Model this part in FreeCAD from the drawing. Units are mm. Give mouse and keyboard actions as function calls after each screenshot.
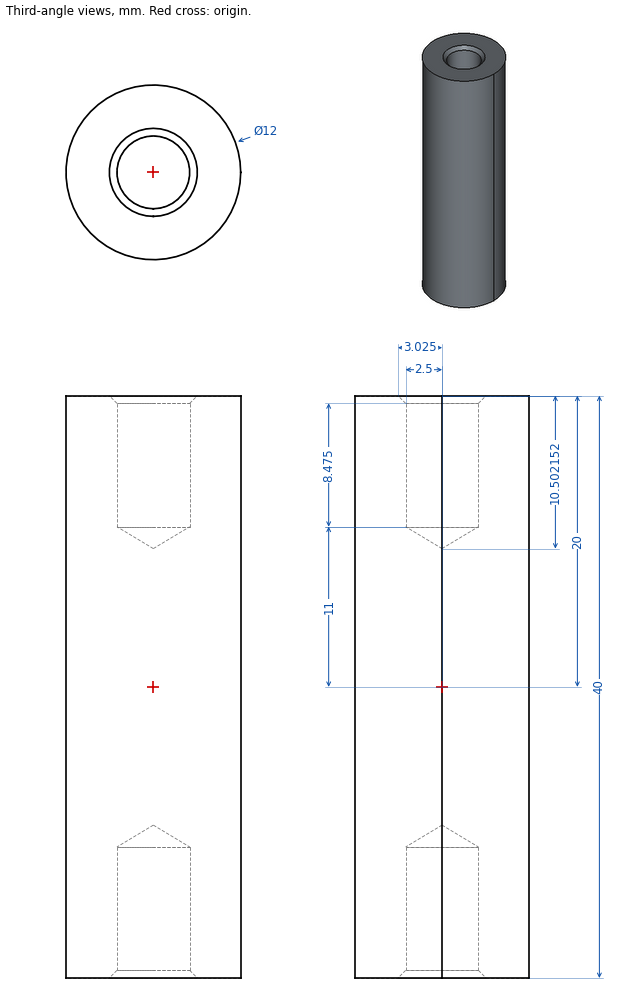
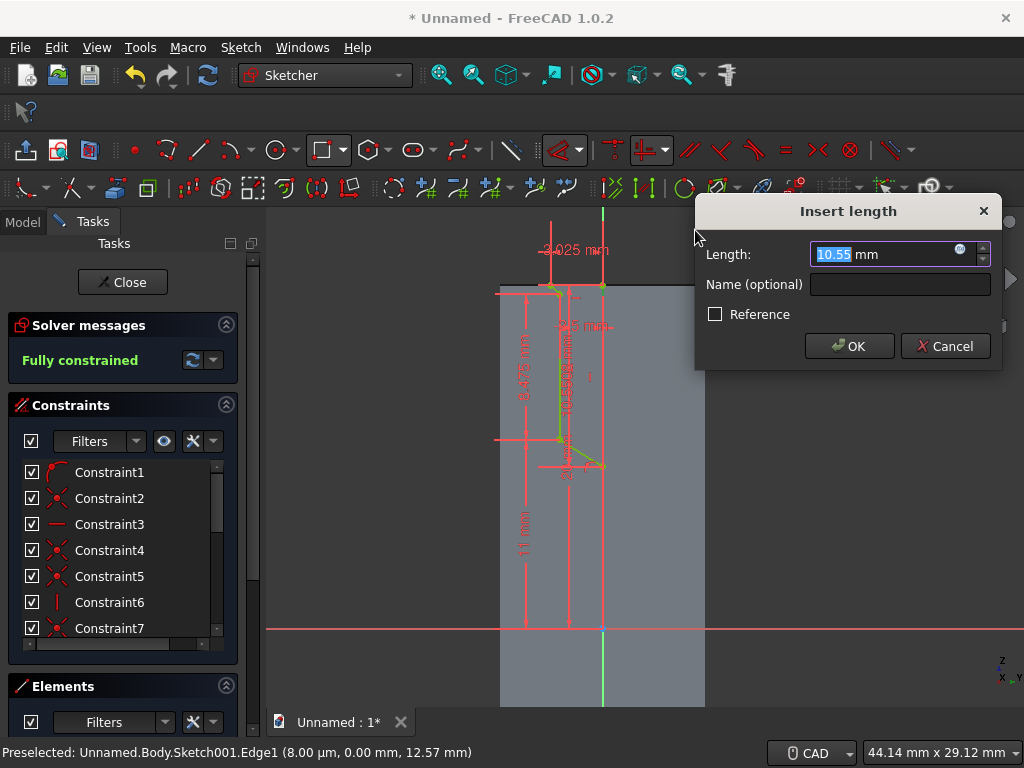
text(10.502152)
key(Return)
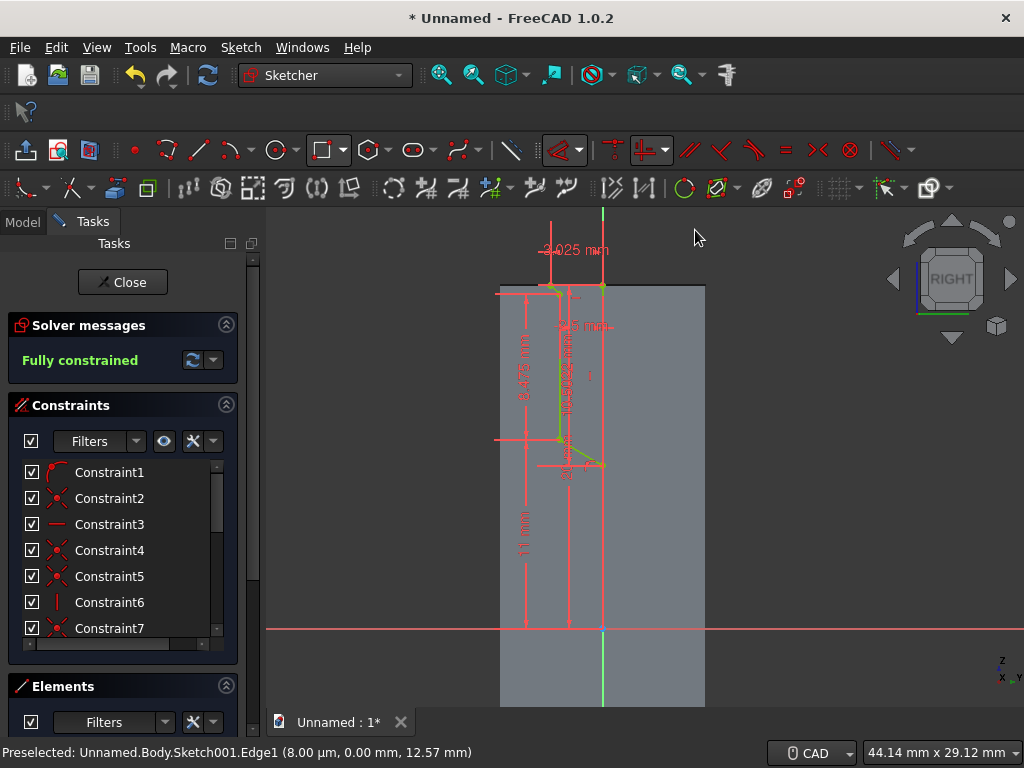
click(123, 282)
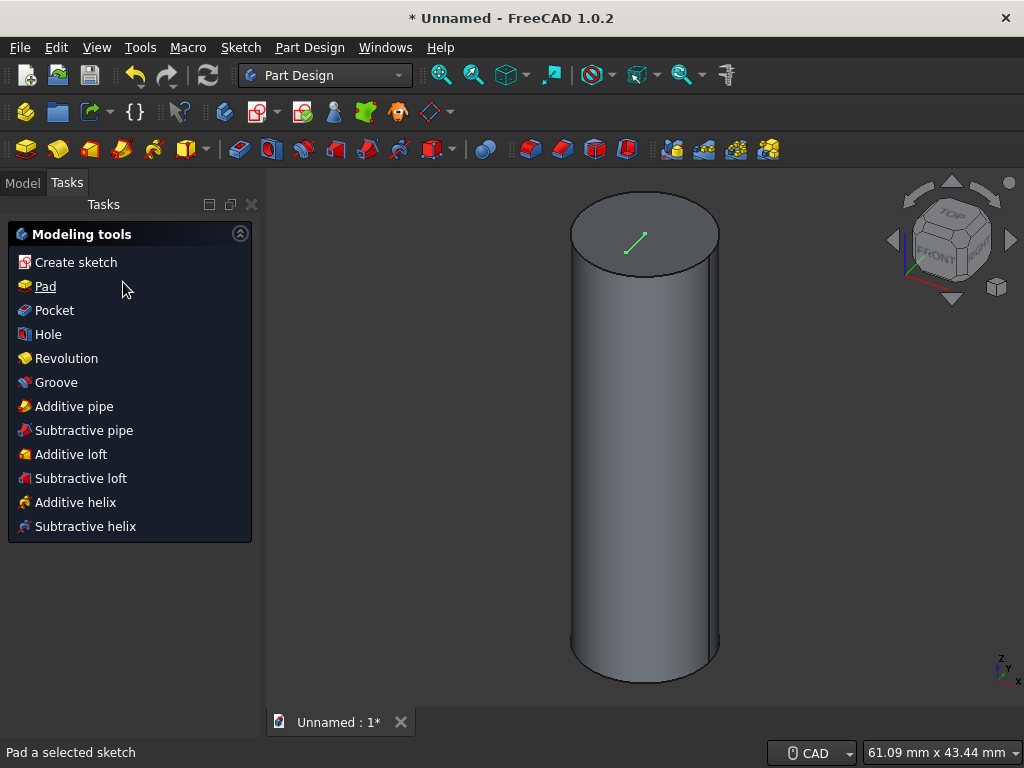
click(304, 150)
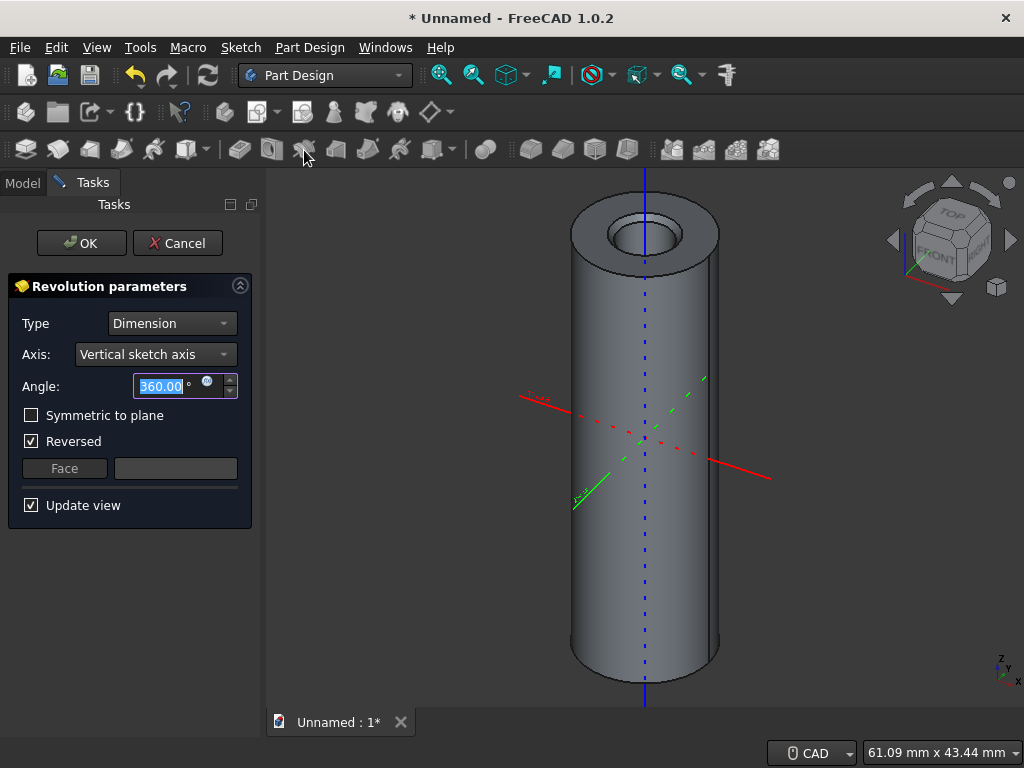
click(82, 243)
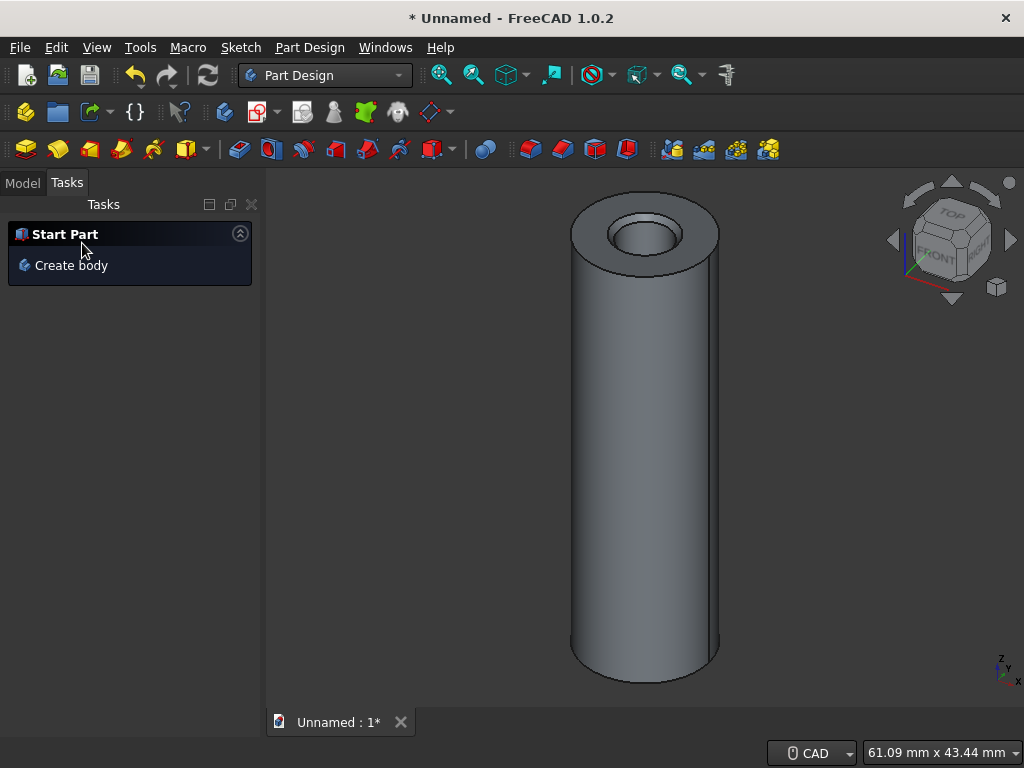
click(23, 182)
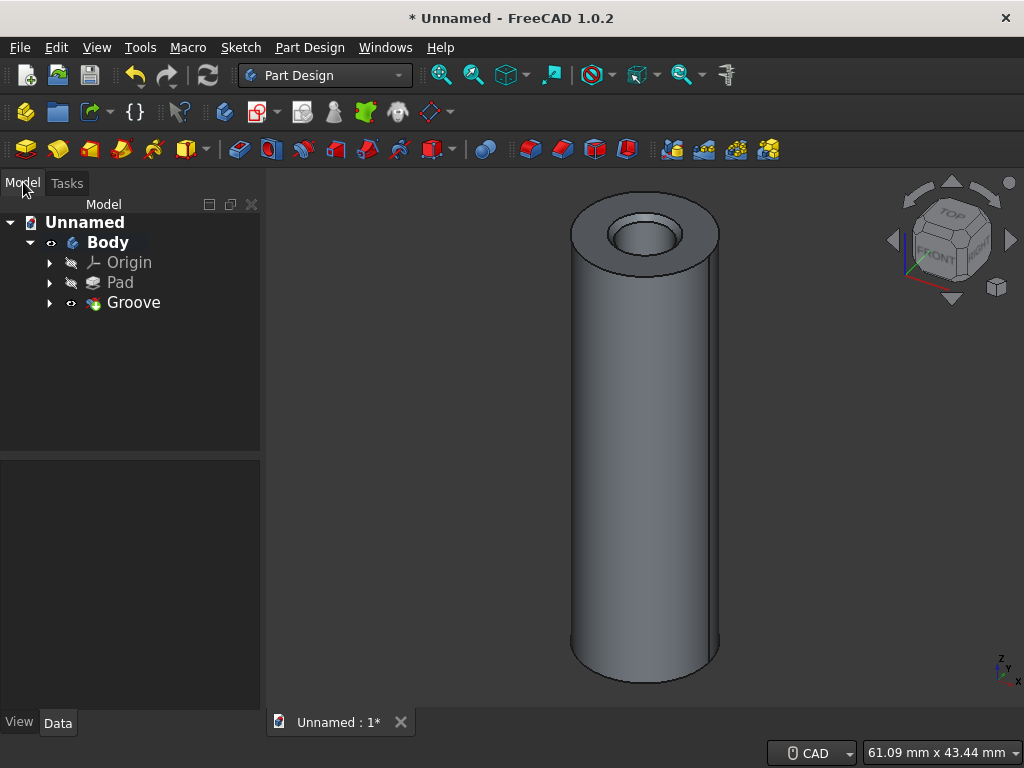
click(116, 303)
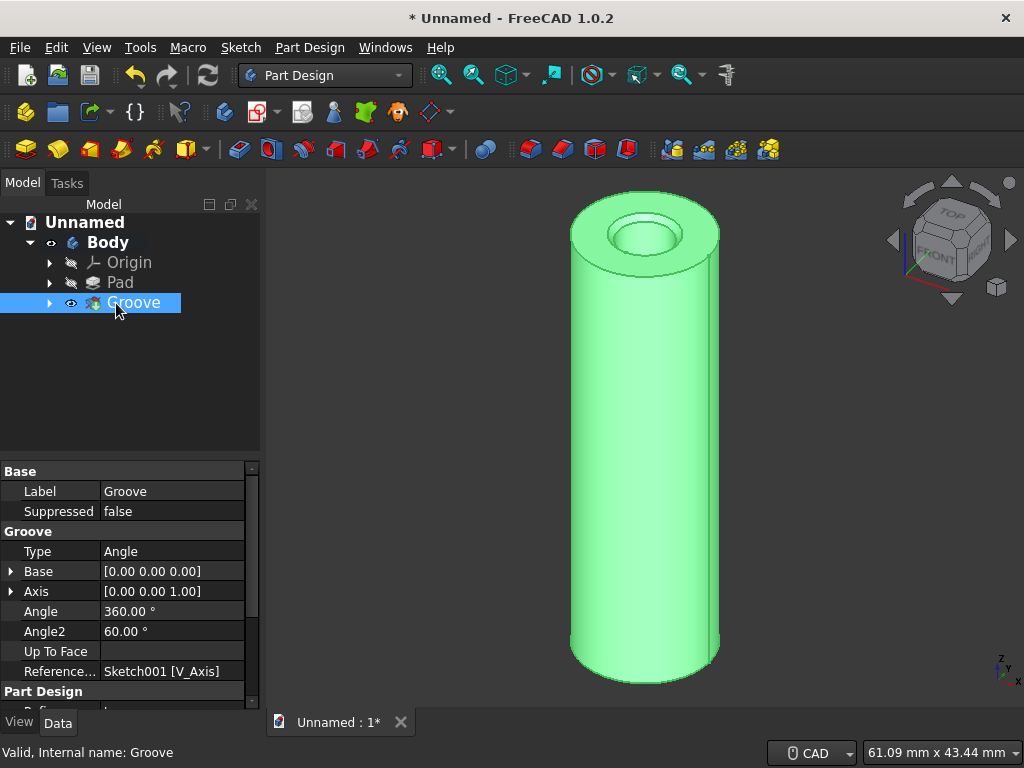
click(672, 150)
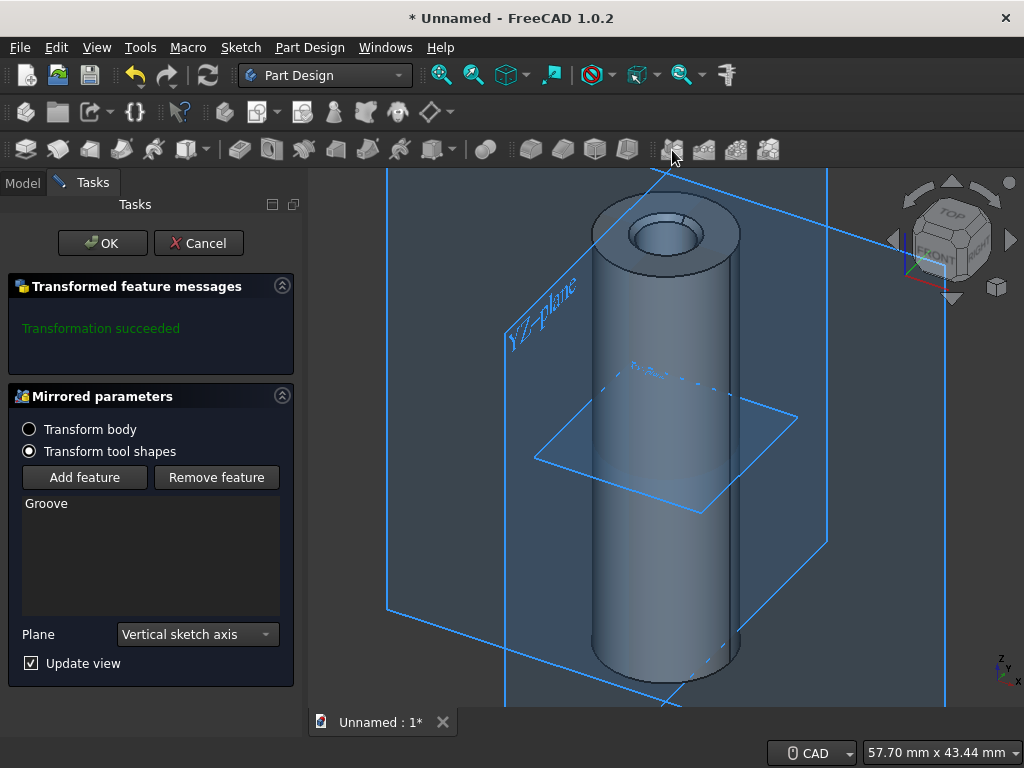
click(198, 634)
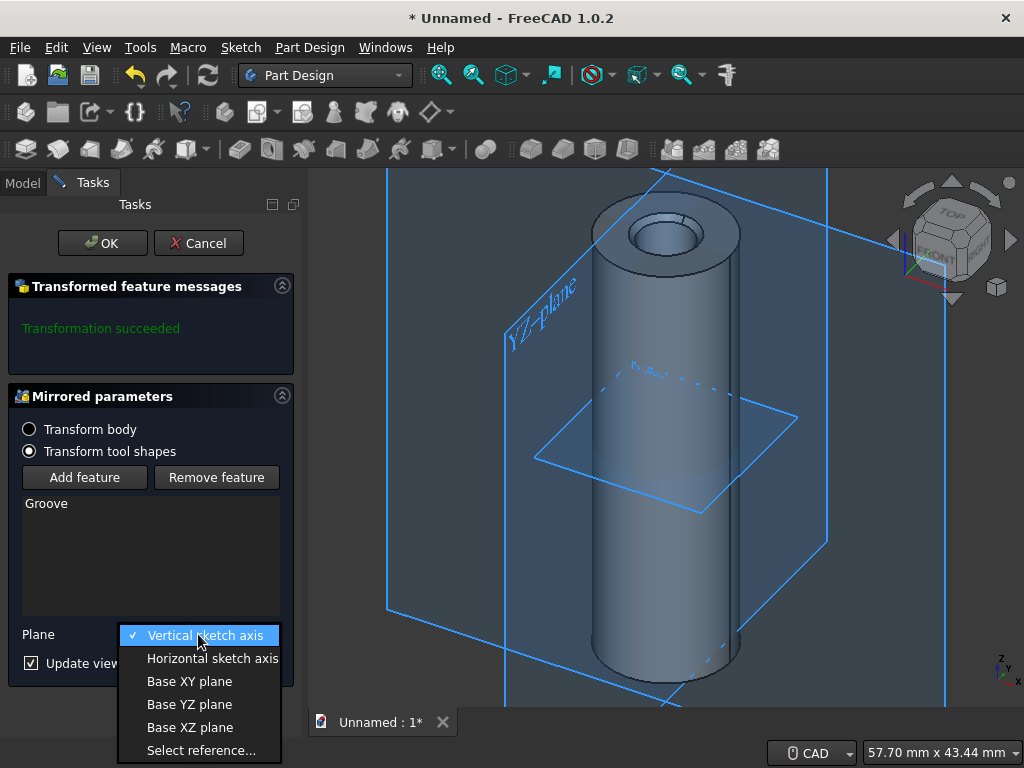
click(198, 682)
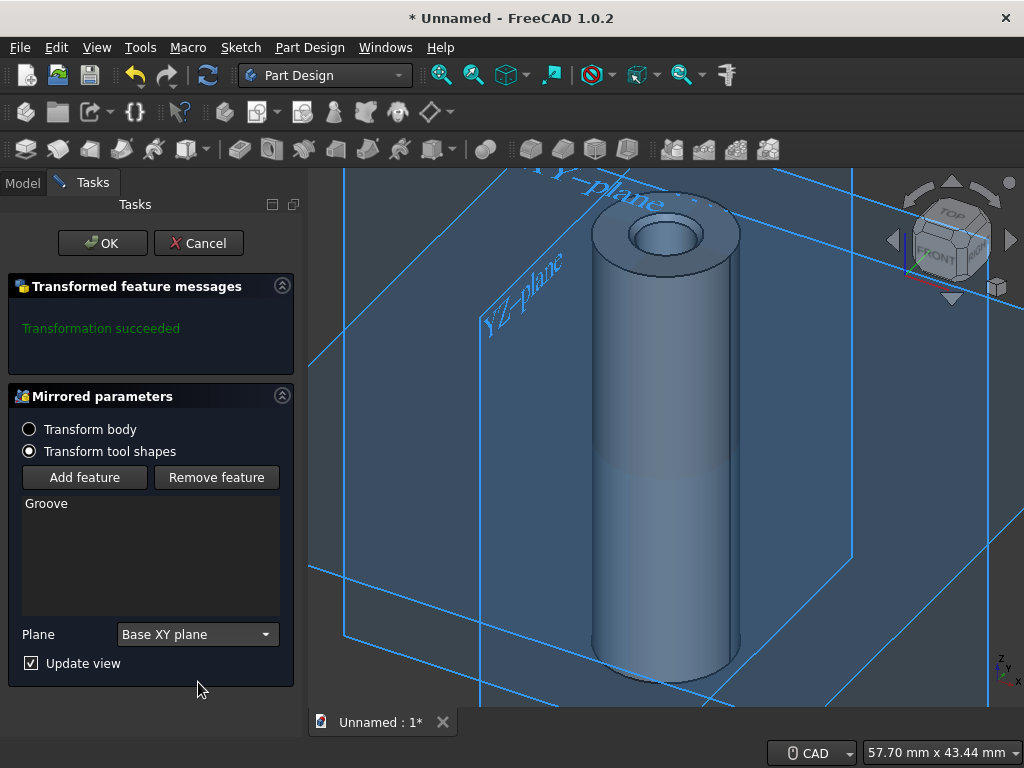
click(103, 243)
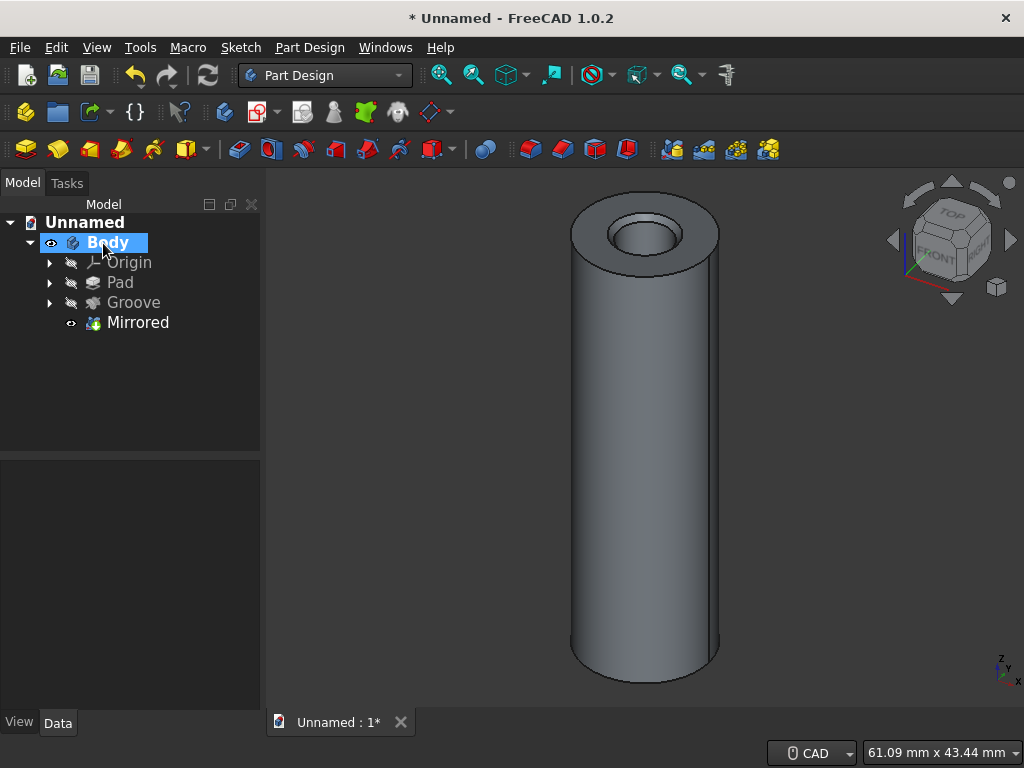
key(0)